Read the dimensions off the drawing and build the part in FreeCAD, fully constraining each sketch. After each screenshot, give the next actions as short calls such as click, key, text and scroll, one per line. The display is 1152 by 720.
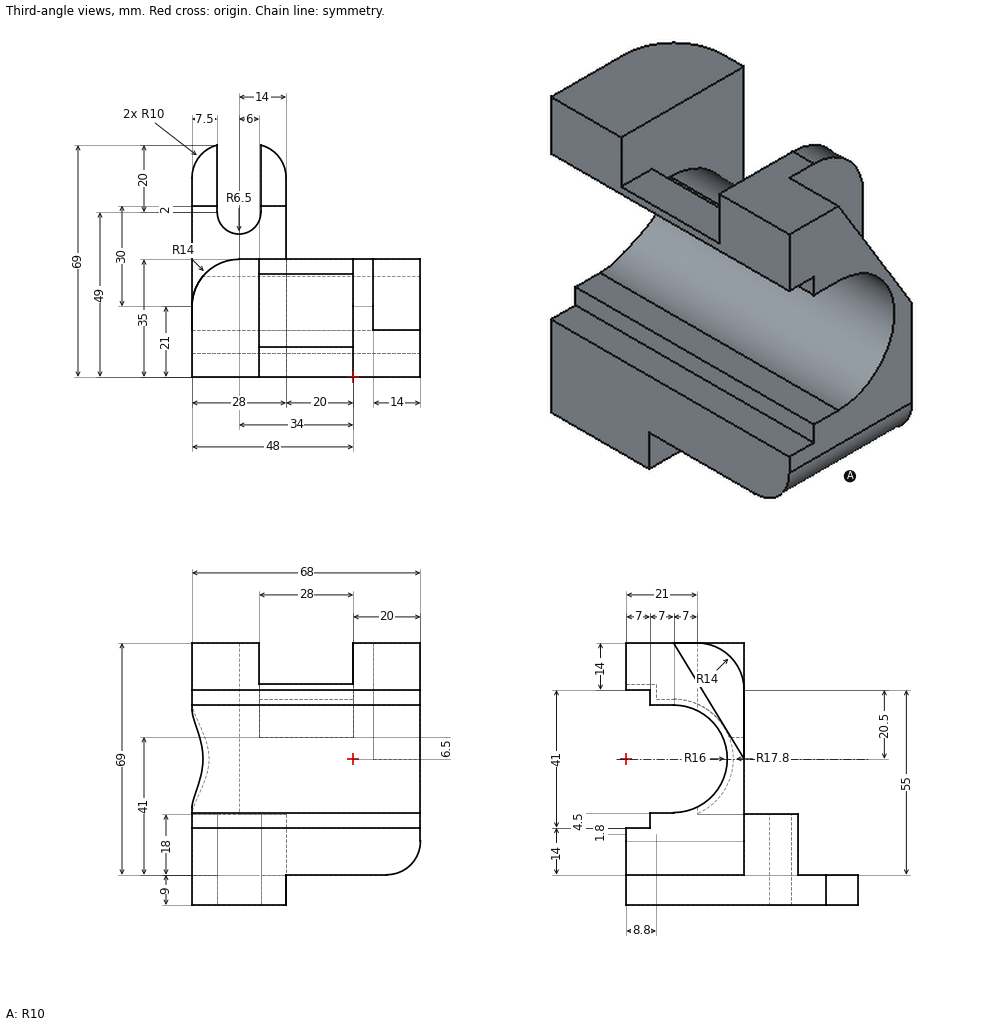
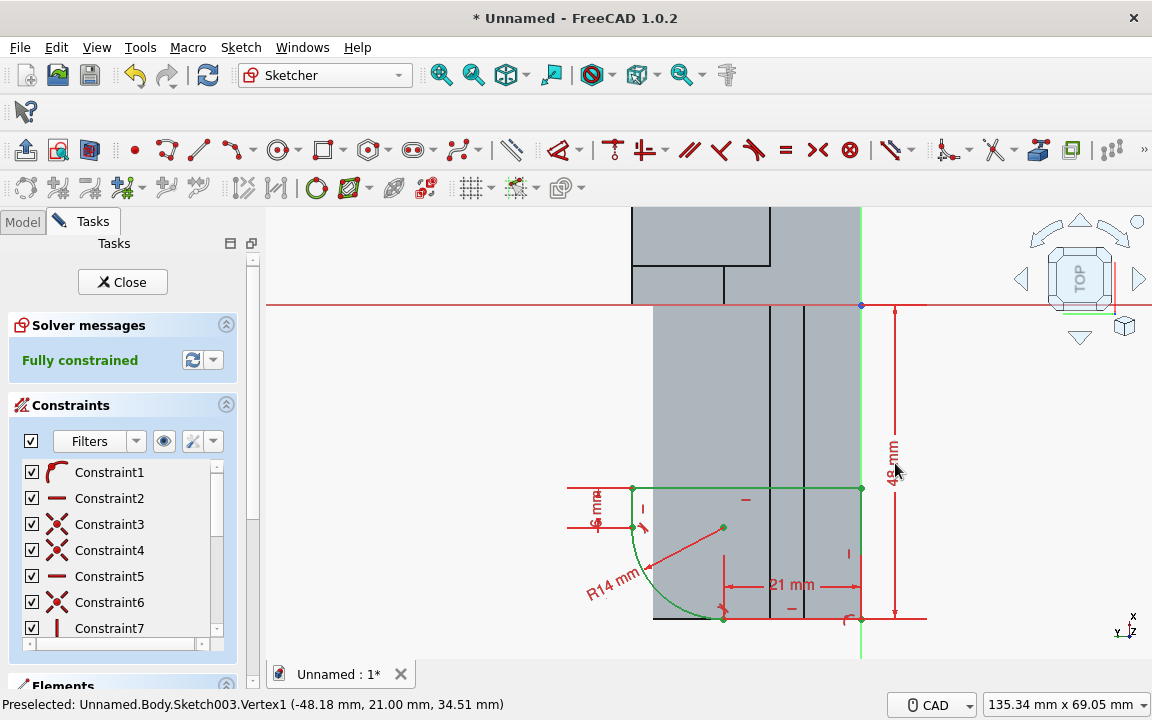
click(123, 282)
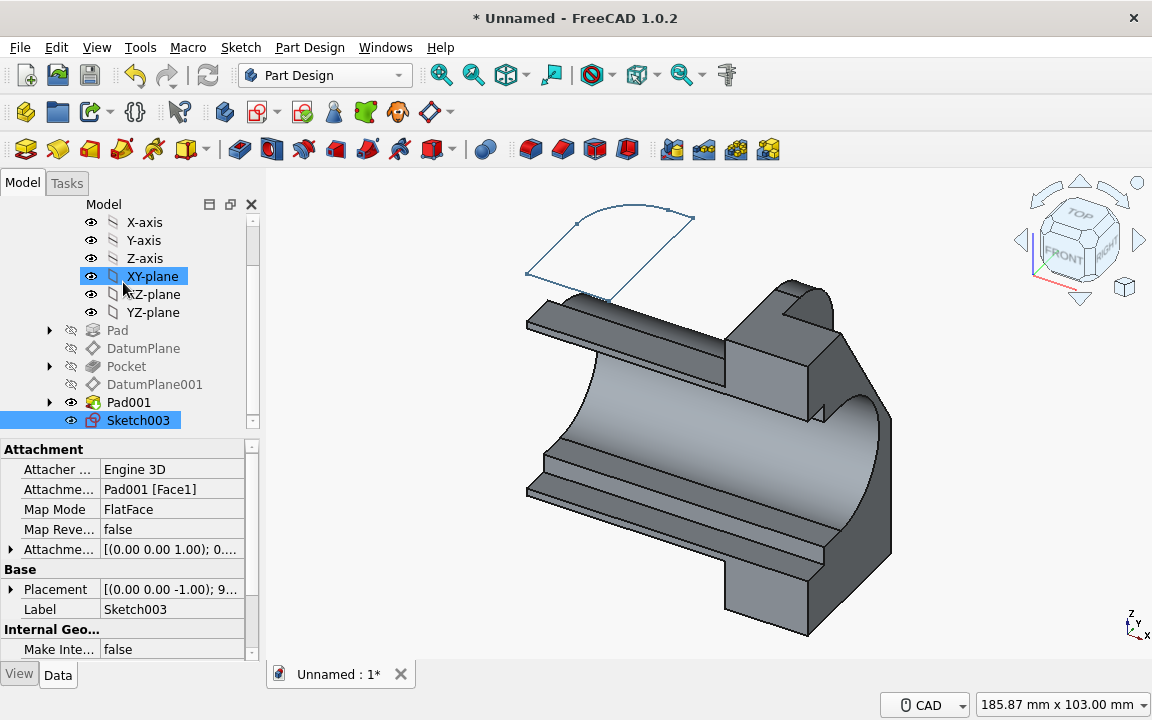
click(26, 150)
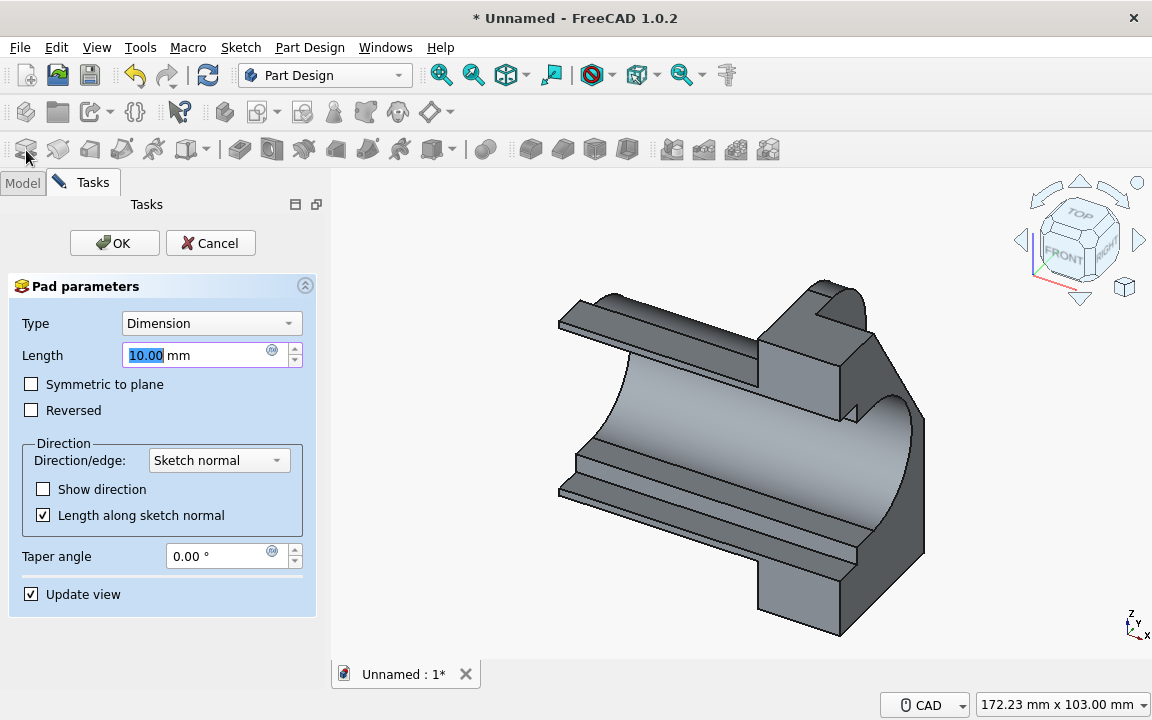
text(69)
key(Tab)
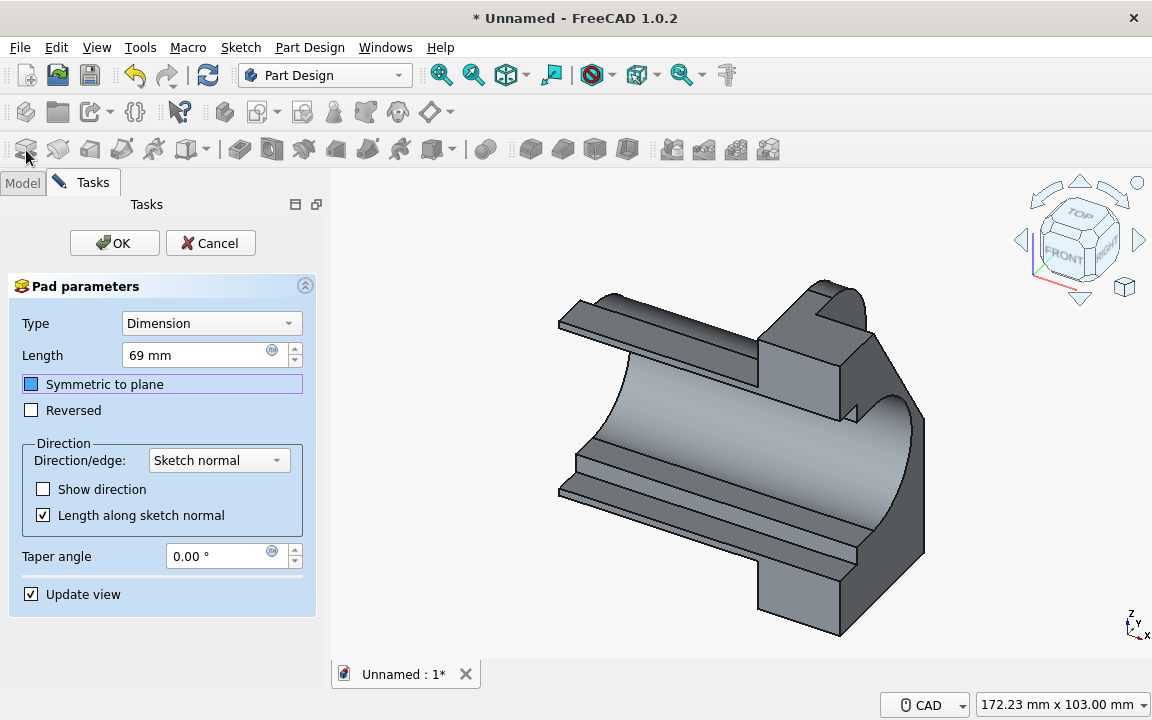
click(30, 410)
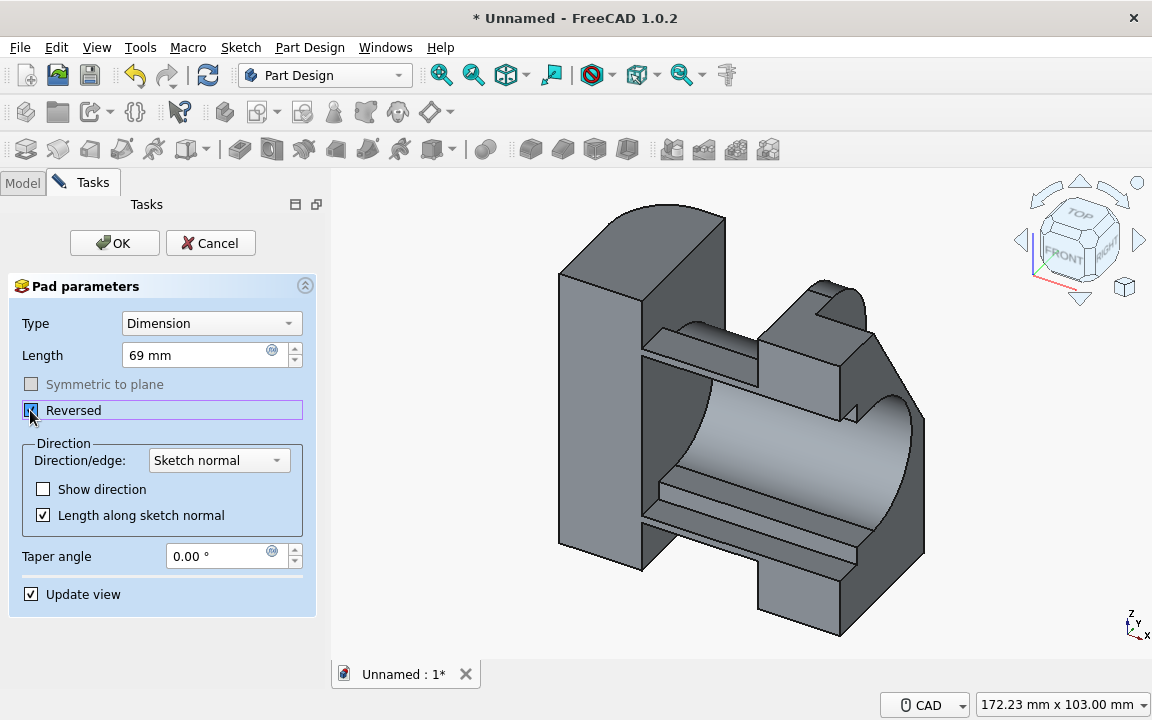
click(115, 243)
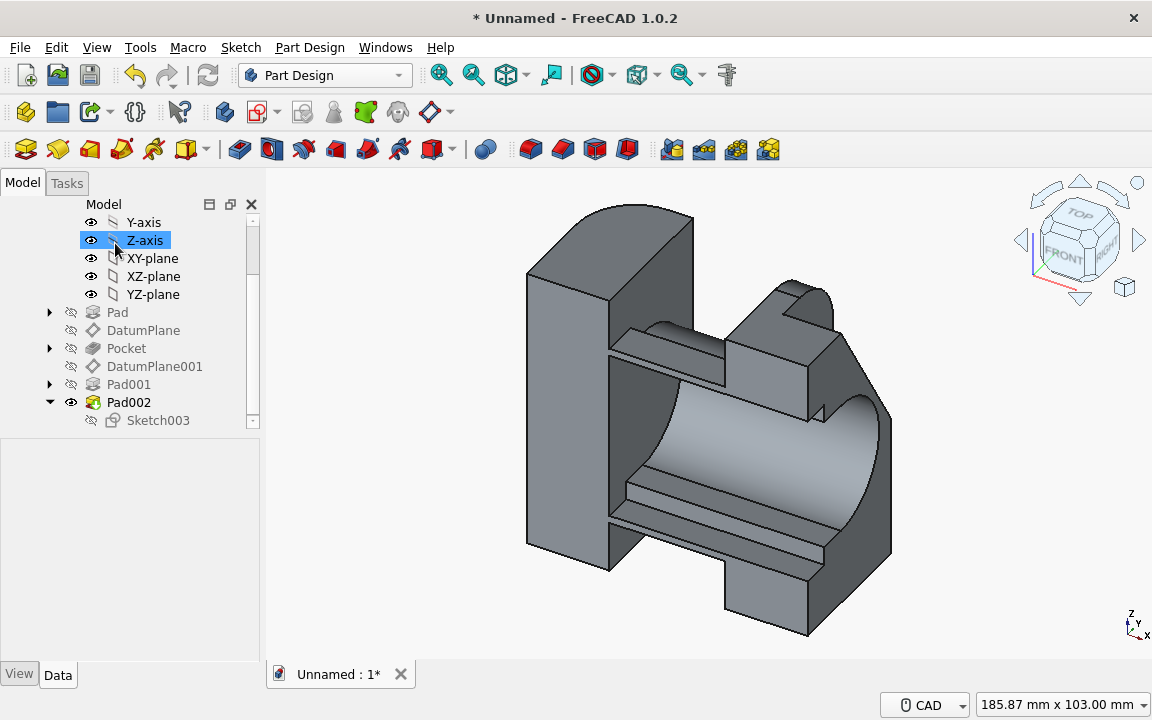
scroll(160, 326, down, 3)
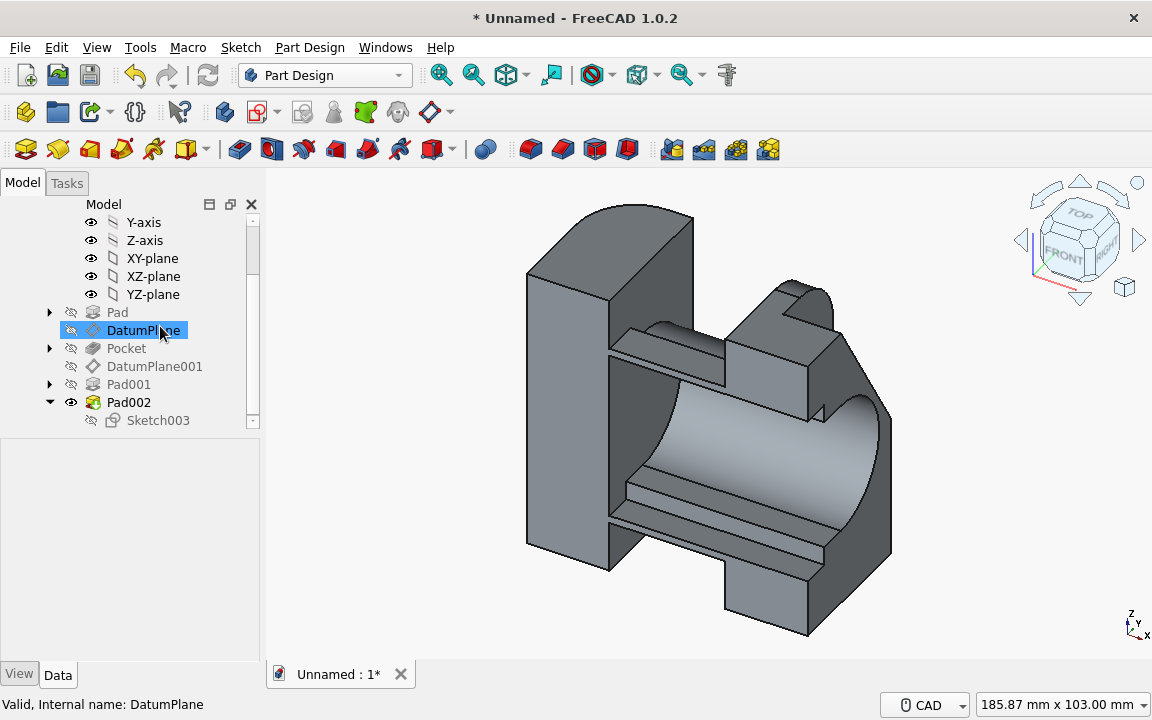
scroll(160, 326, up, 15)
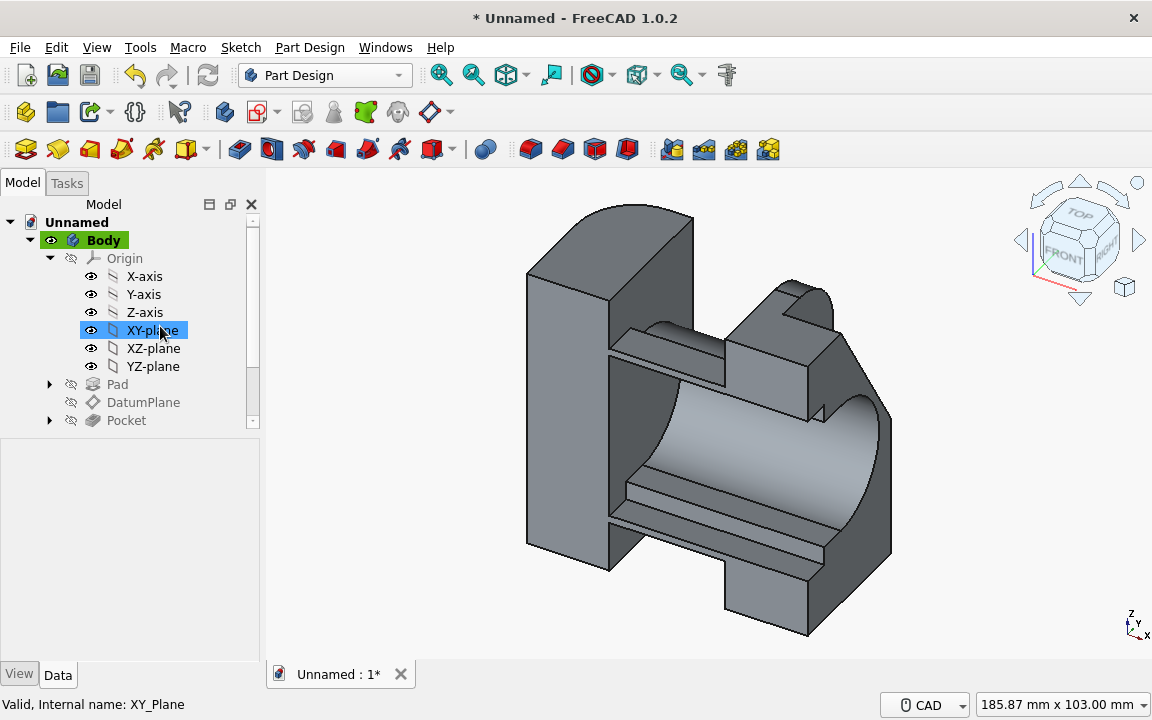
click(136, 366)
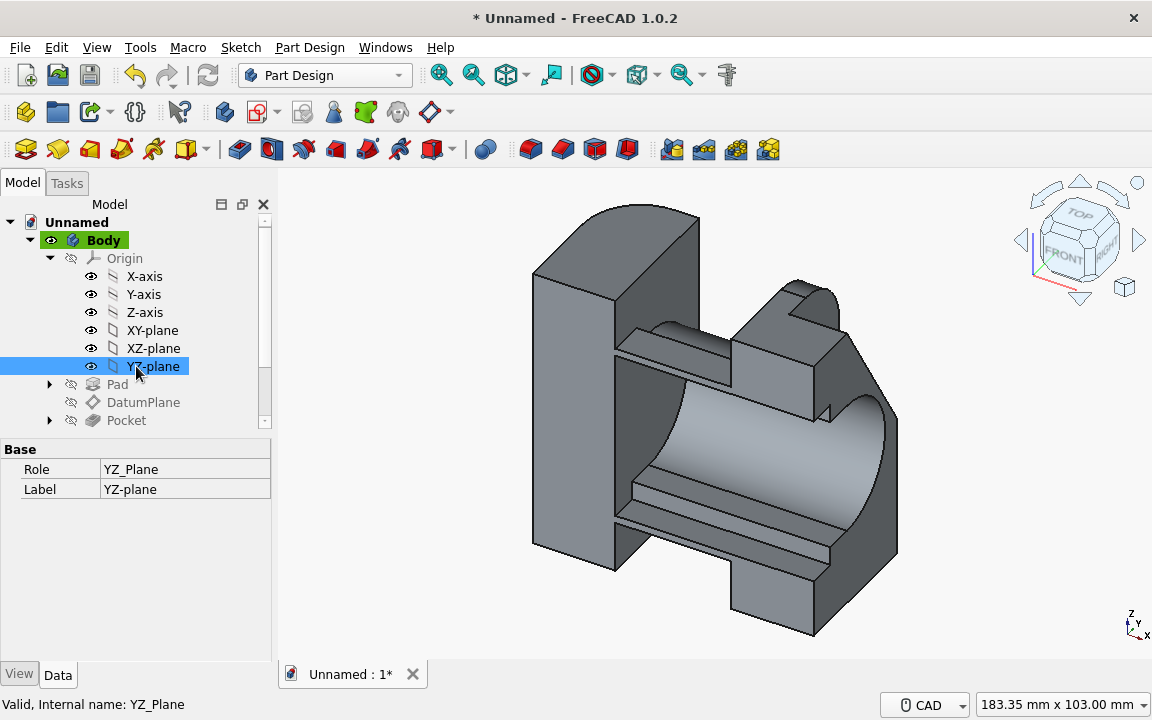
click(430, 112)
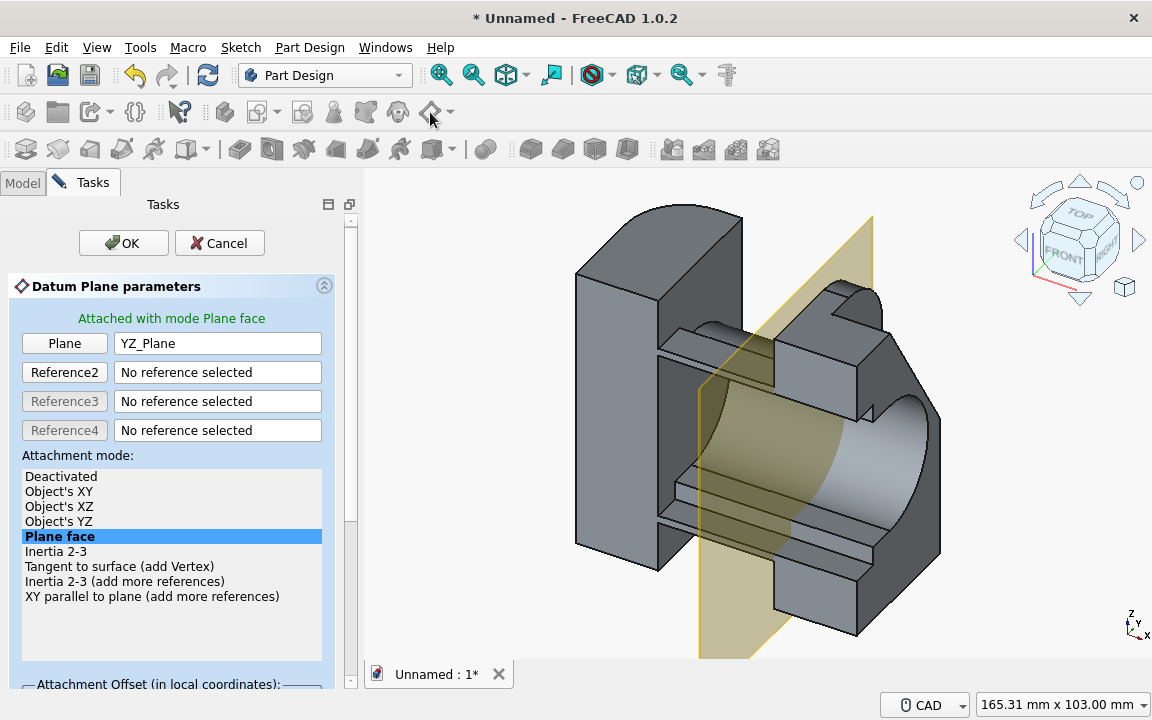
scroll(351, 451, down, 3)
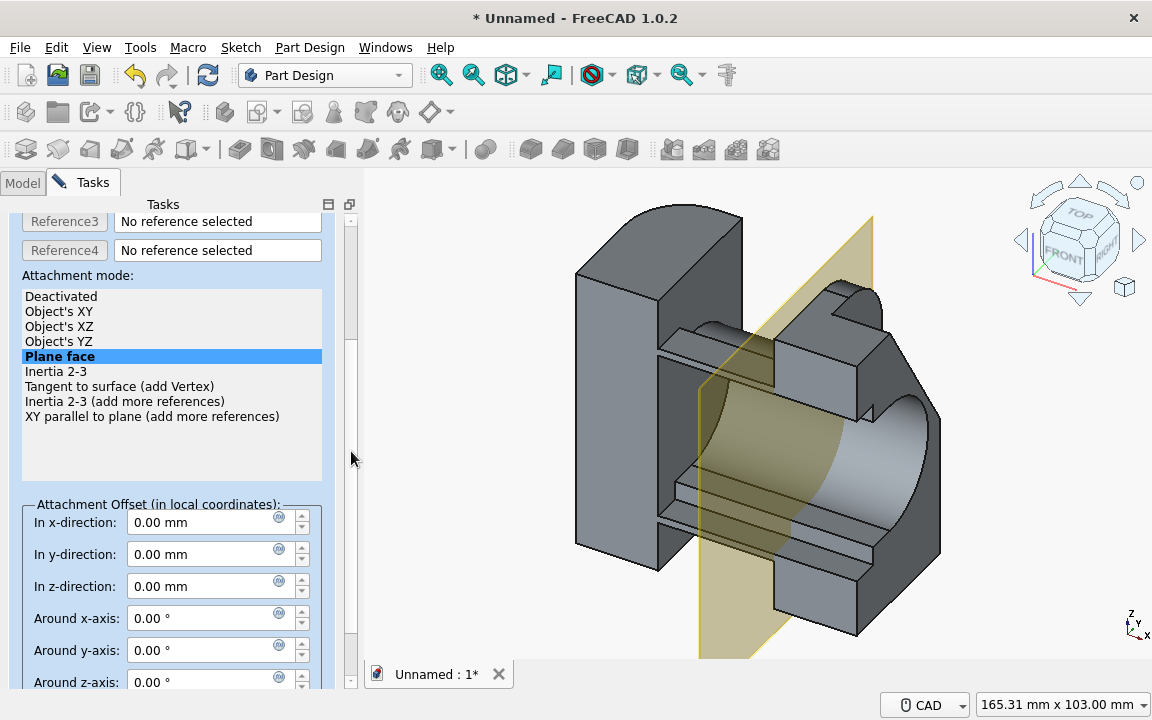
triple_click(210, 586)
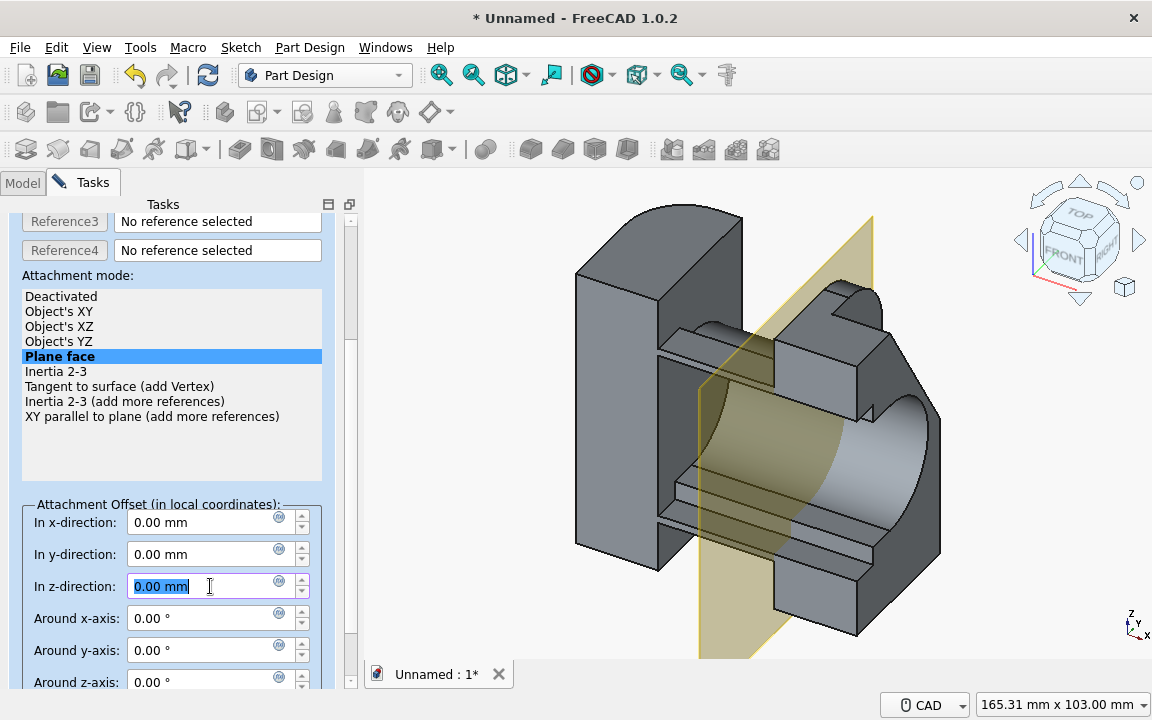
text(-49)
key(Tab)